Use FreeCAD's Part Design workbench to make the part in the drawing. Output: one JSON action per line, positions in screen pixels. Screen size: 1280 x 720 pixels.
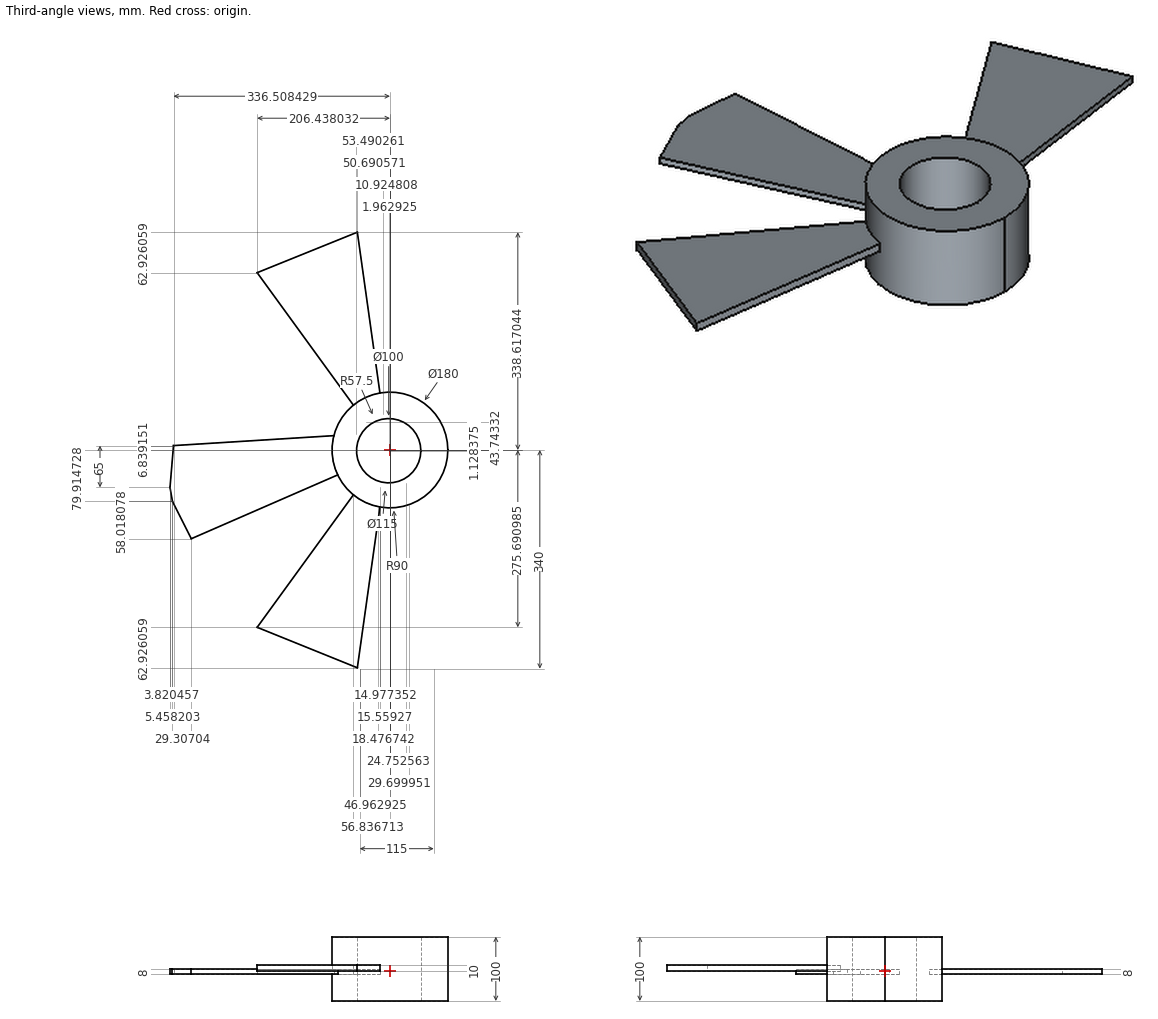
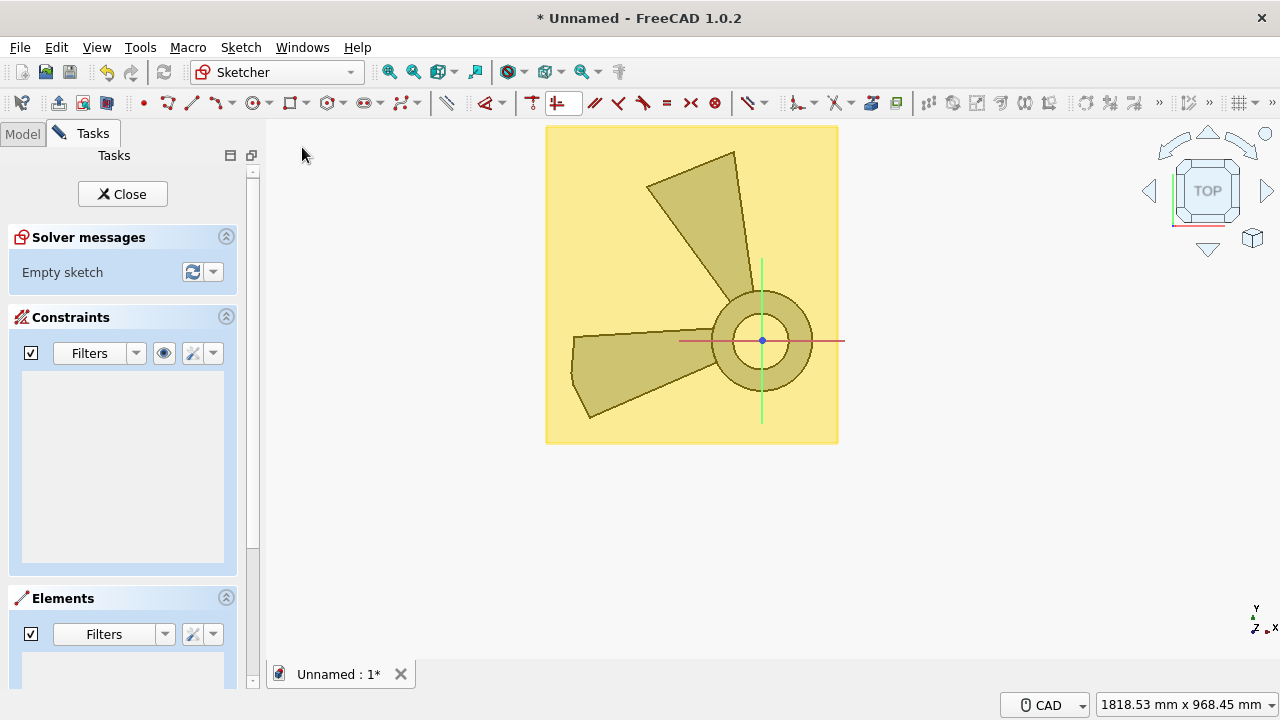
{"action": "scroll", "coordinate": [704, 491], "scroll_direction": "up", "scroll_amount": 3}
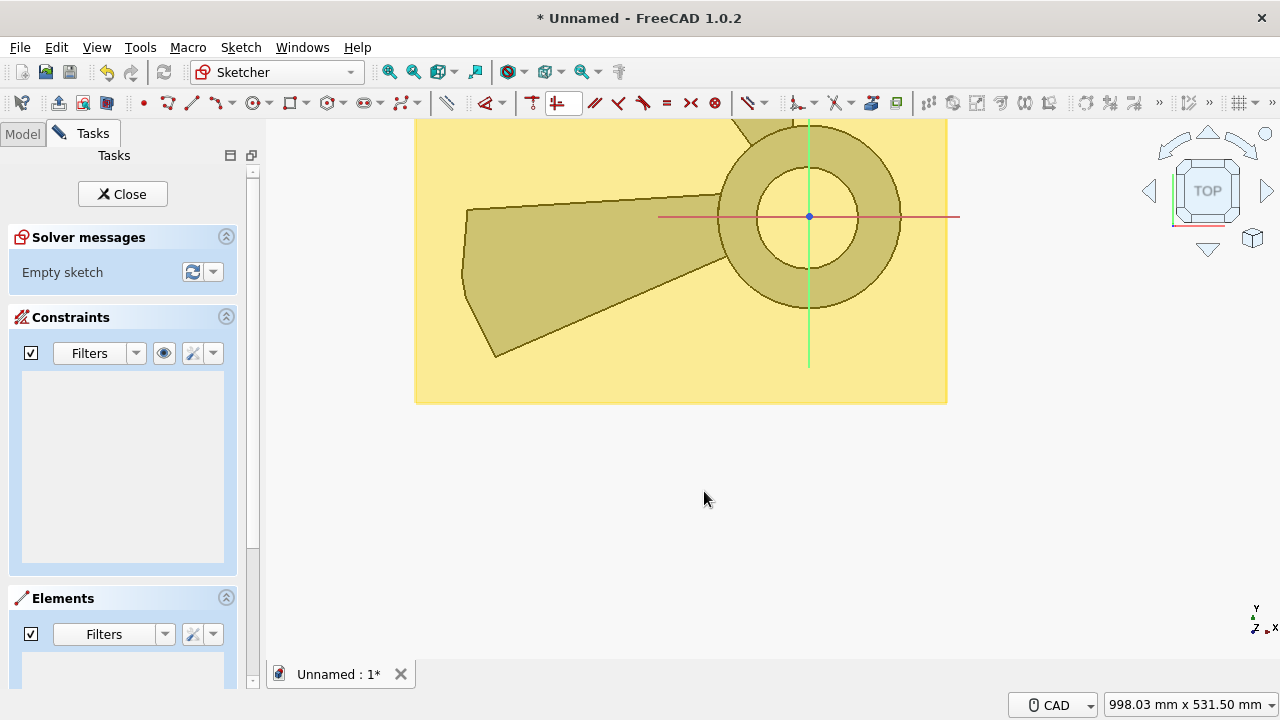
{"action": "left_click", "coordinate": [168, 104]}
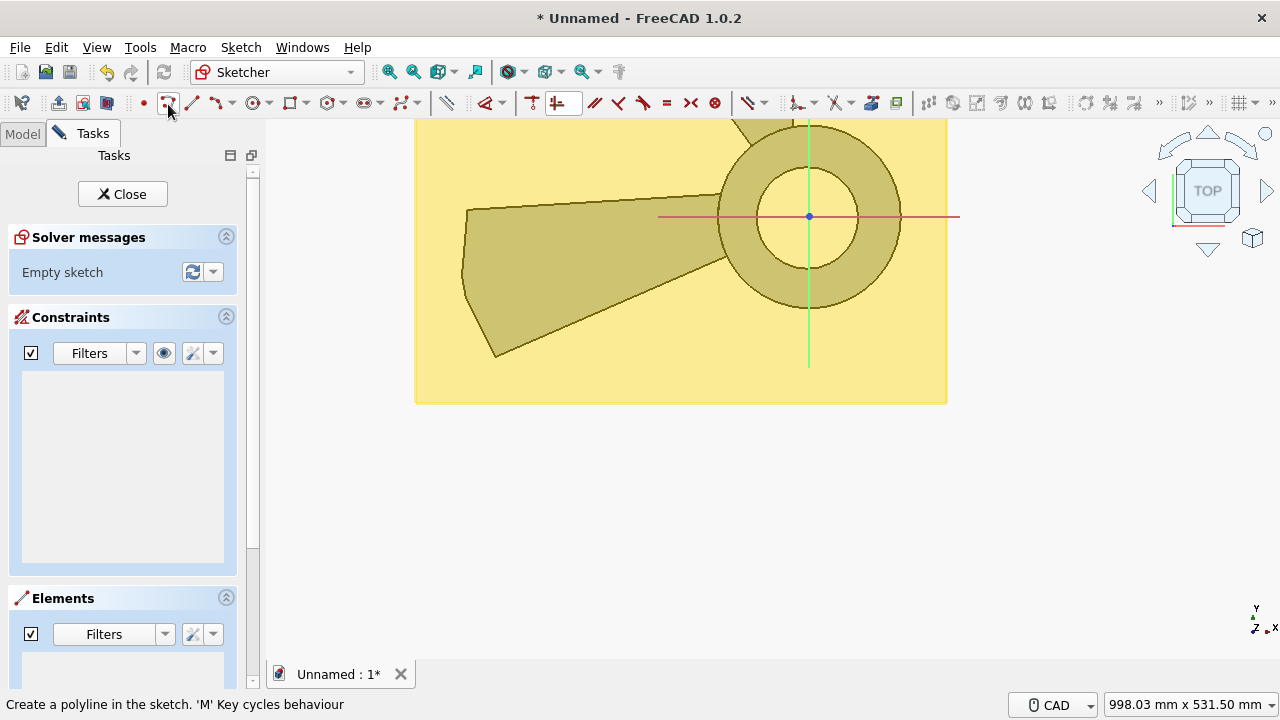
{"action": "left_click", "coordinate": [752, 288]}
{"action": "left_click", "coordinate": [600, 497]}
{"action": "left_click", "coordinate": [758, 561]}
{"action": "left_click", "coordinate": [794, 307]}
{"action": "right_click", "coordinate": [794, 307]}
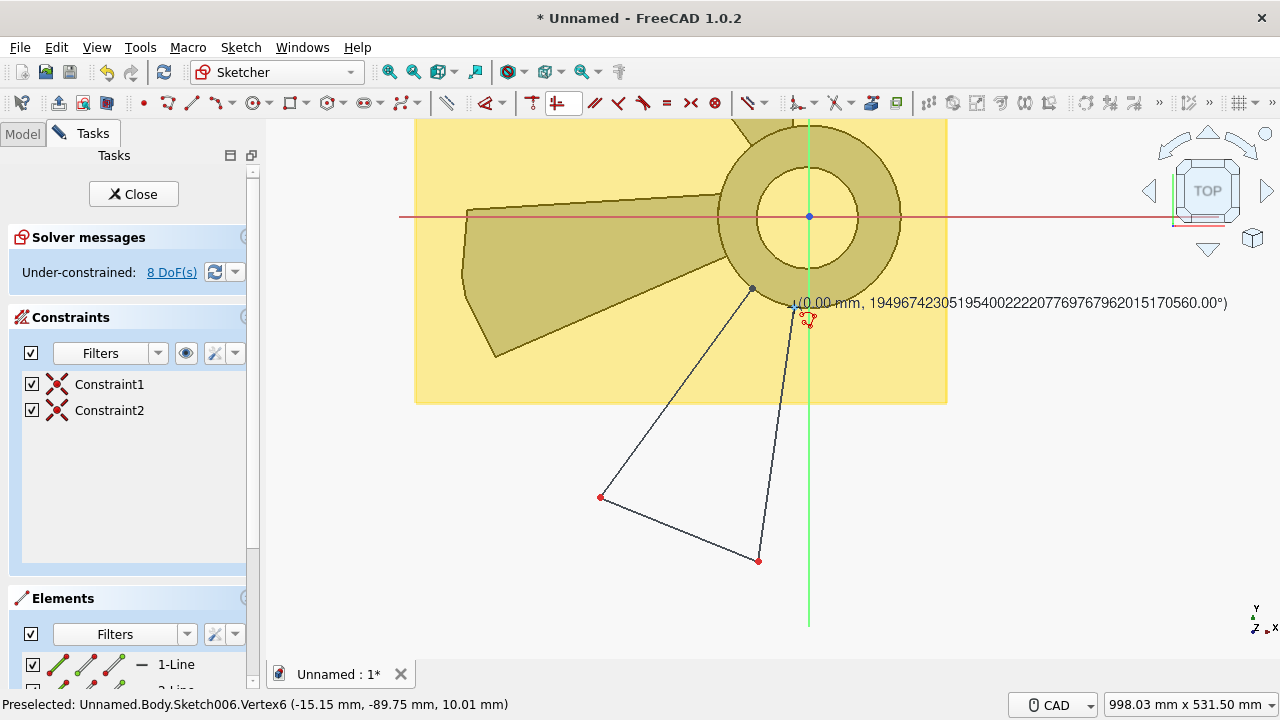
{"action": "left_click", "coordinate": [216, 104]}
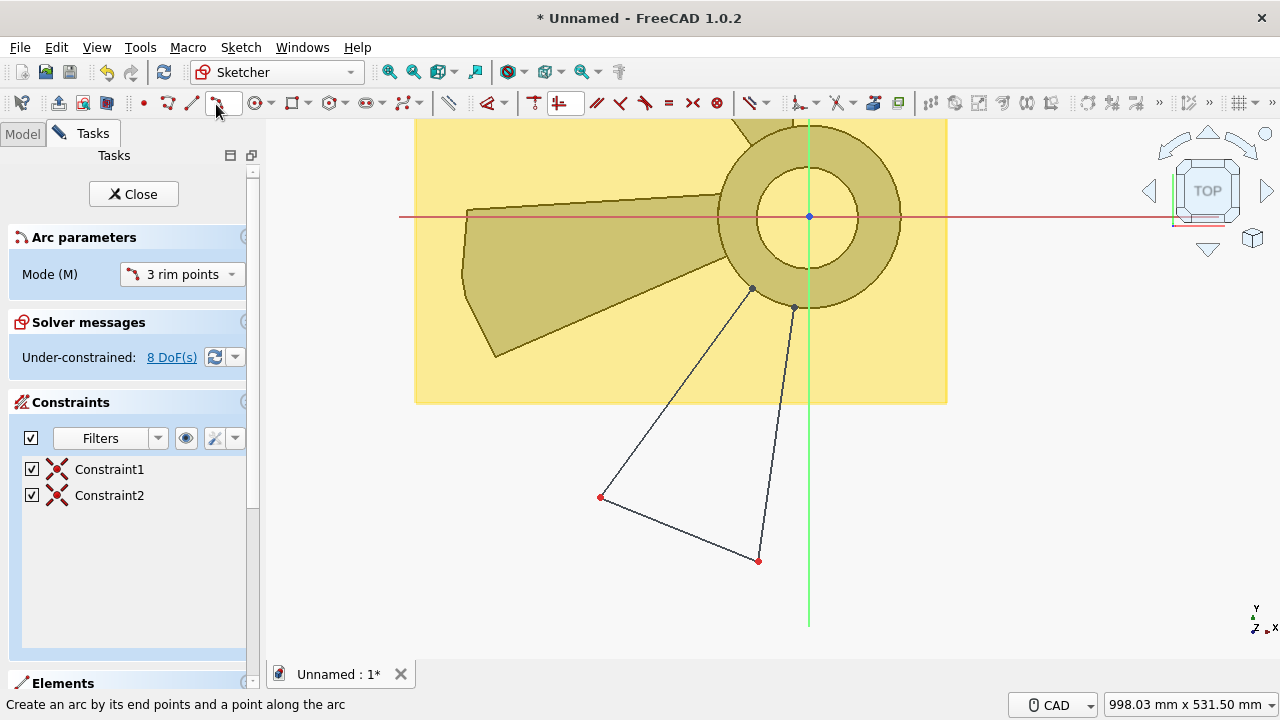
{"action": "left_click", "coordinate": [794, 308]}
{"action": "left_click", "coordinate": [752, 289]}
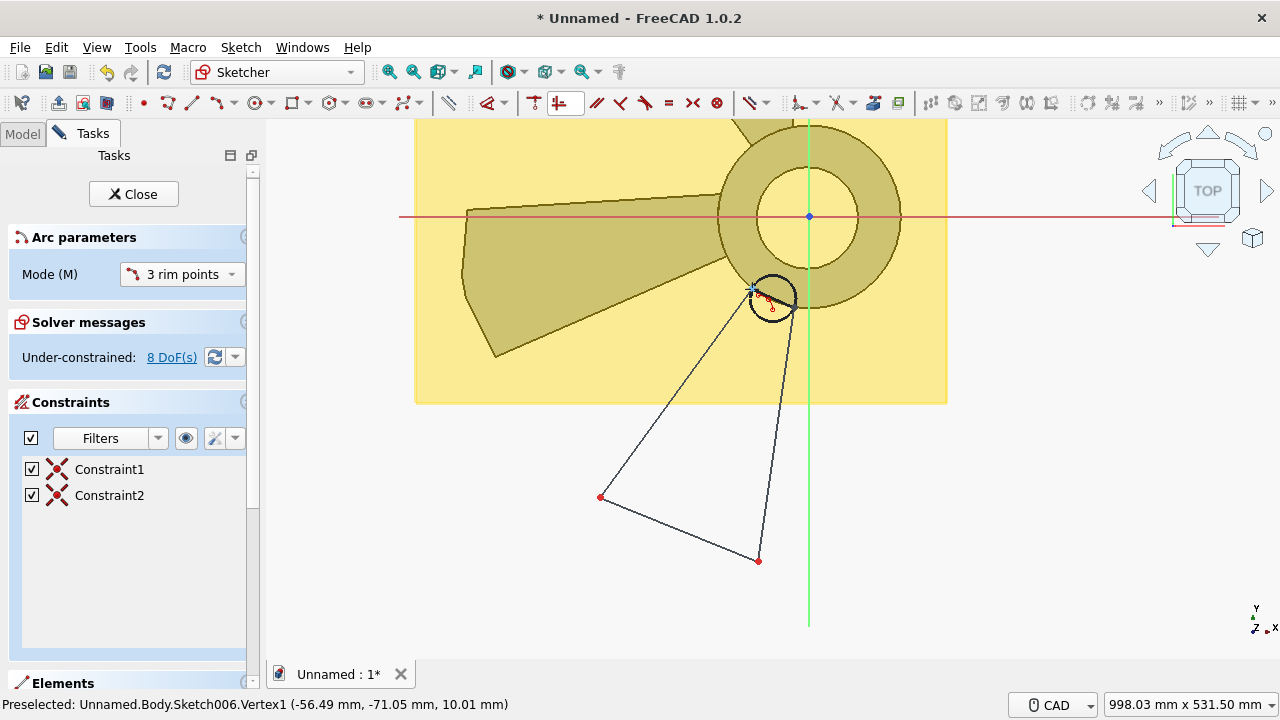
{"action": "scroll", "coordinate": [771, 300], "scroll_direction": "up", "scroll_amount": 9}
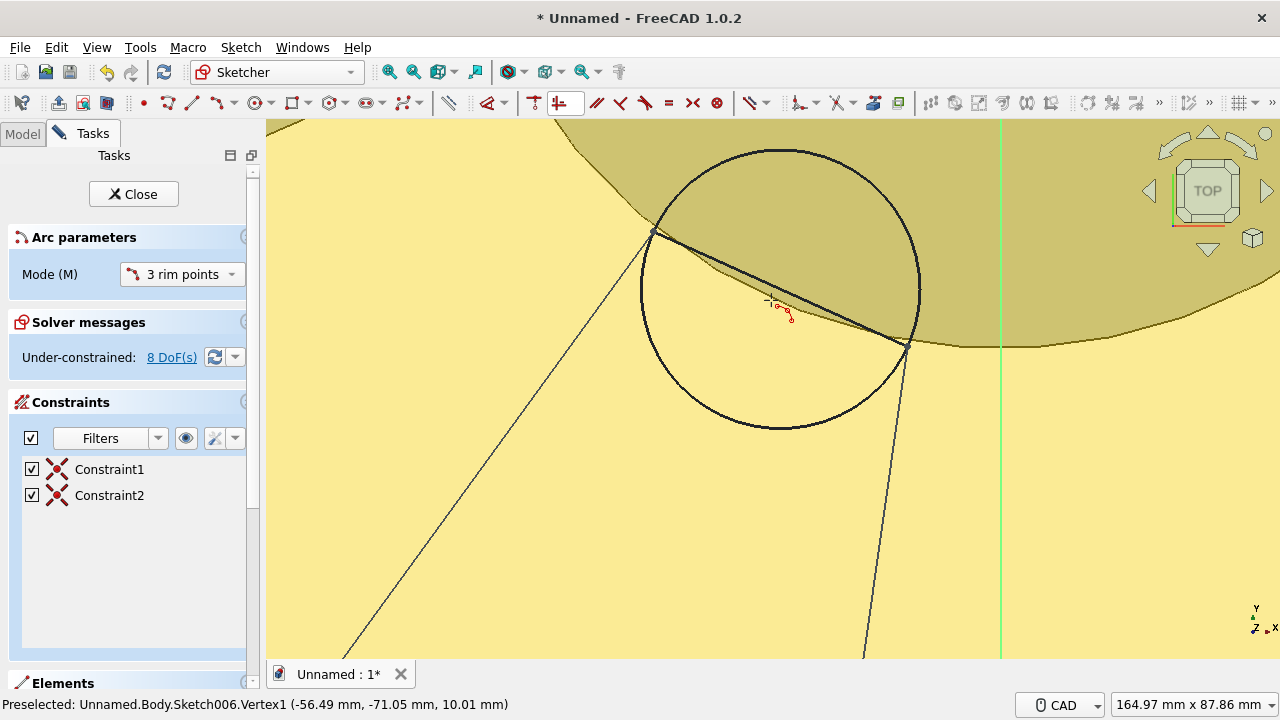
{"action": "left_click", "coordinate": [771, 298]}
{"action": "key", "text": "Escape"}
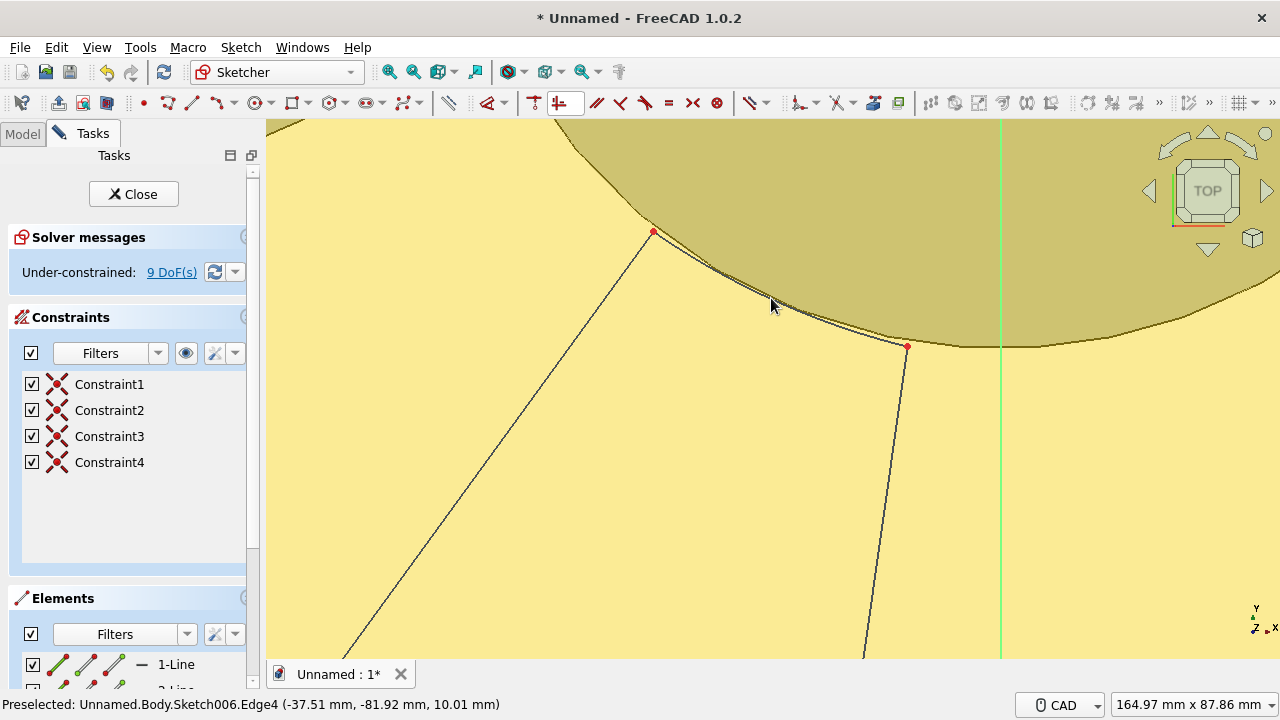
{"action": "scroll", "coordinate": [771, 301], "scroll_direction": "down", "scroll_amount": 9}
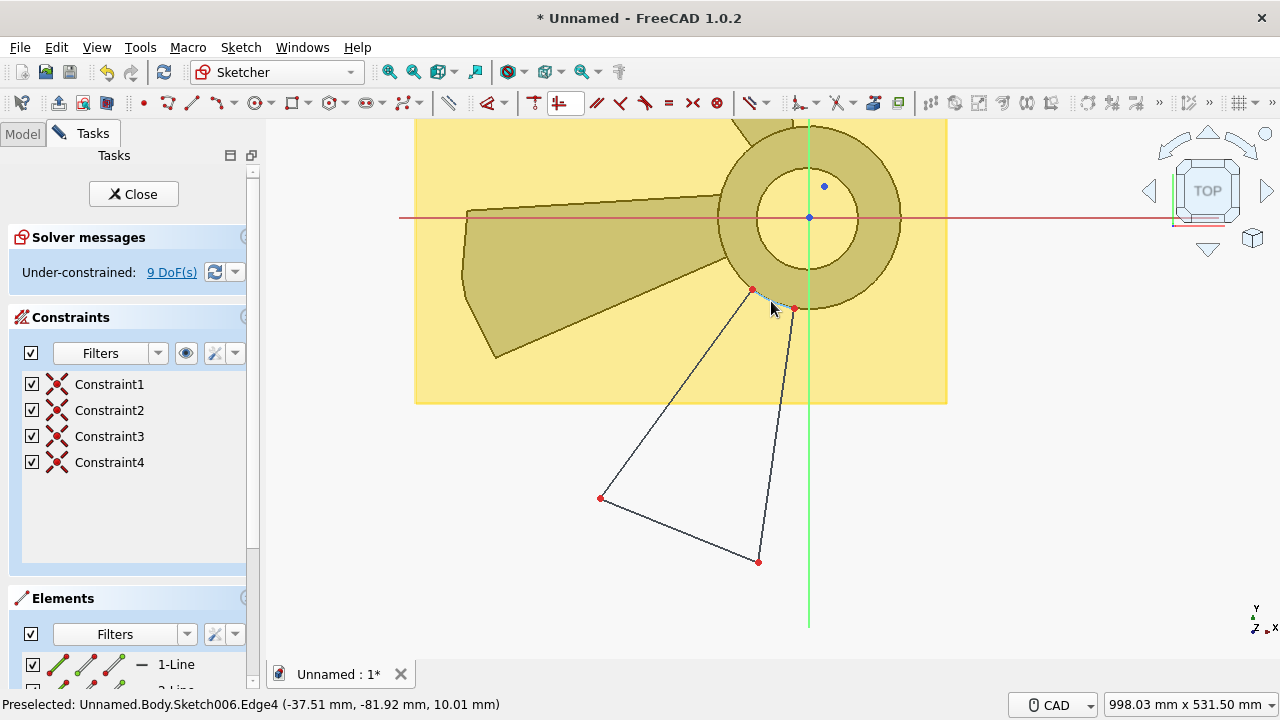
{"action": "left_click_drag", "start_coordinate": [799, 177], "coordinate": [834, 228]}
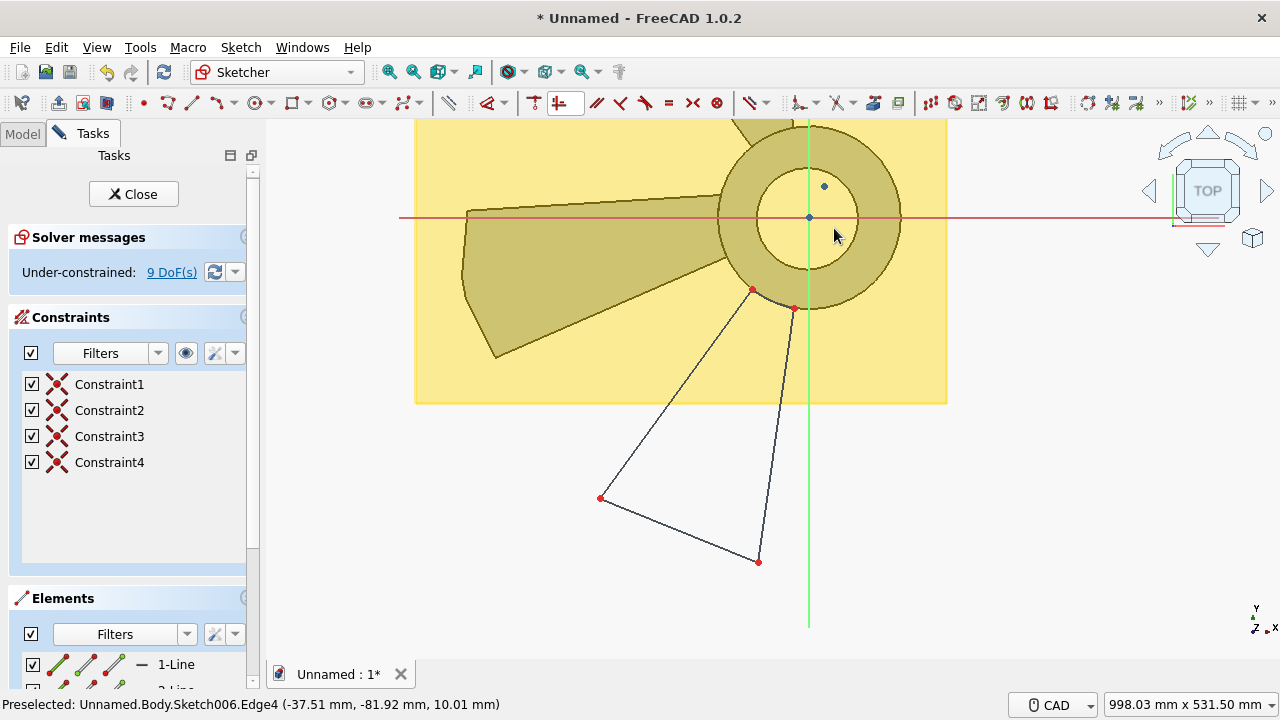
{"action": "left_click", "coordinate": [534, 104]}